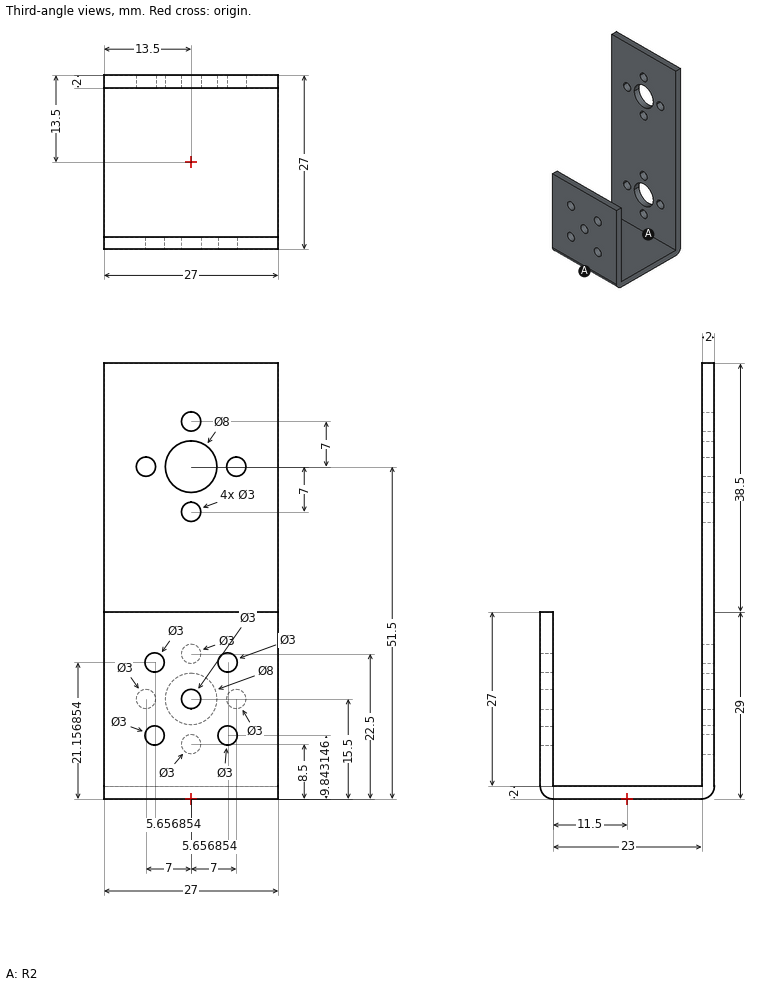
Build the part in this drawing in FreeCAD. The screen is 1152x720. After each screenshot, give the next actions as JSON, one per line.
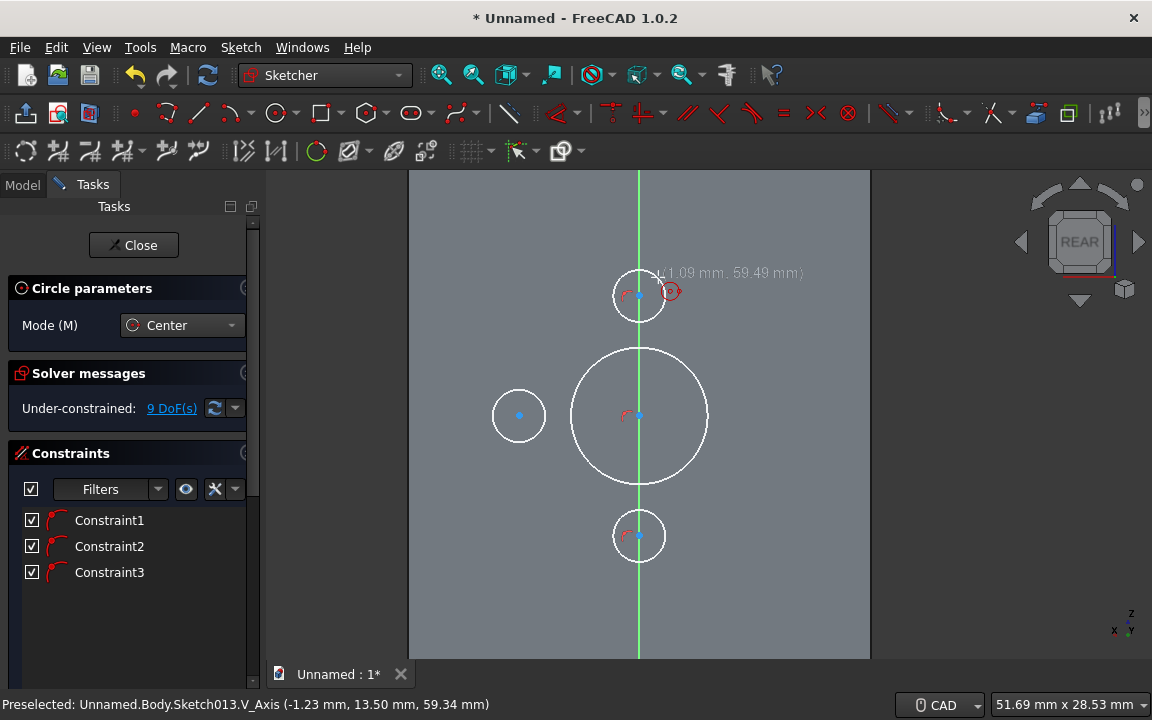
{"action": "left_click", "coordinate": [759, 415]}
{"action": "left_click", "coordinate": [777, 397]}
{"action": "key", "text": "Escape"}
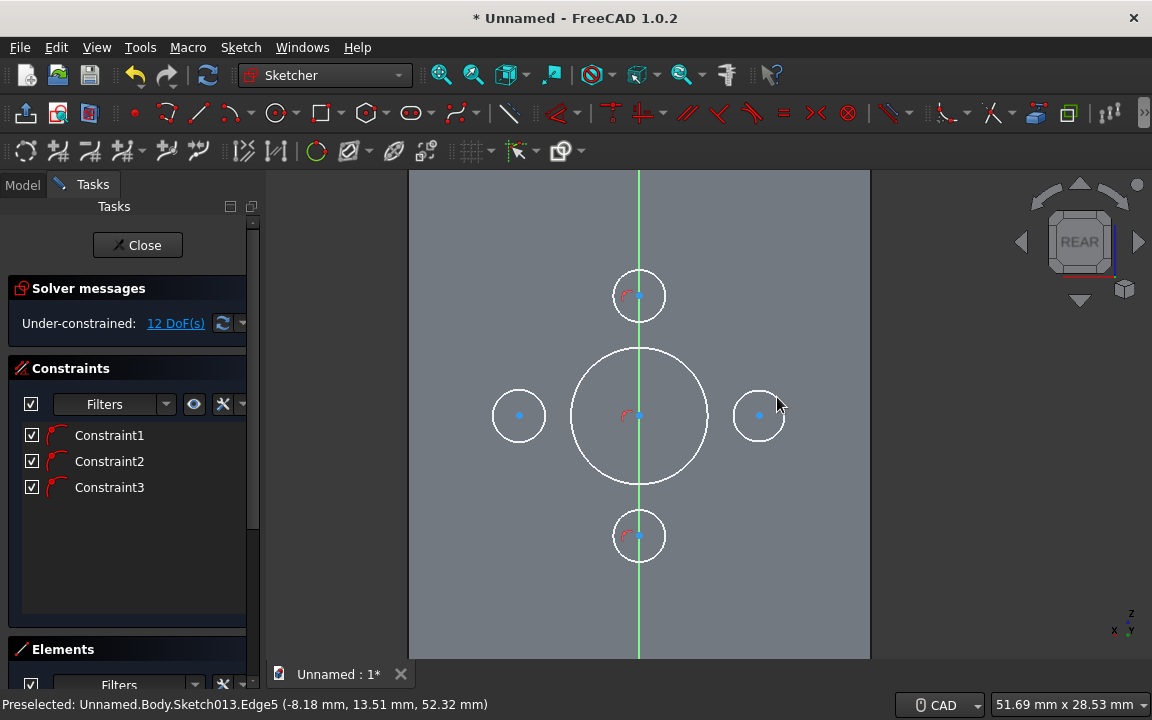
{"action": "left_click", "coordinate": [658, 518]}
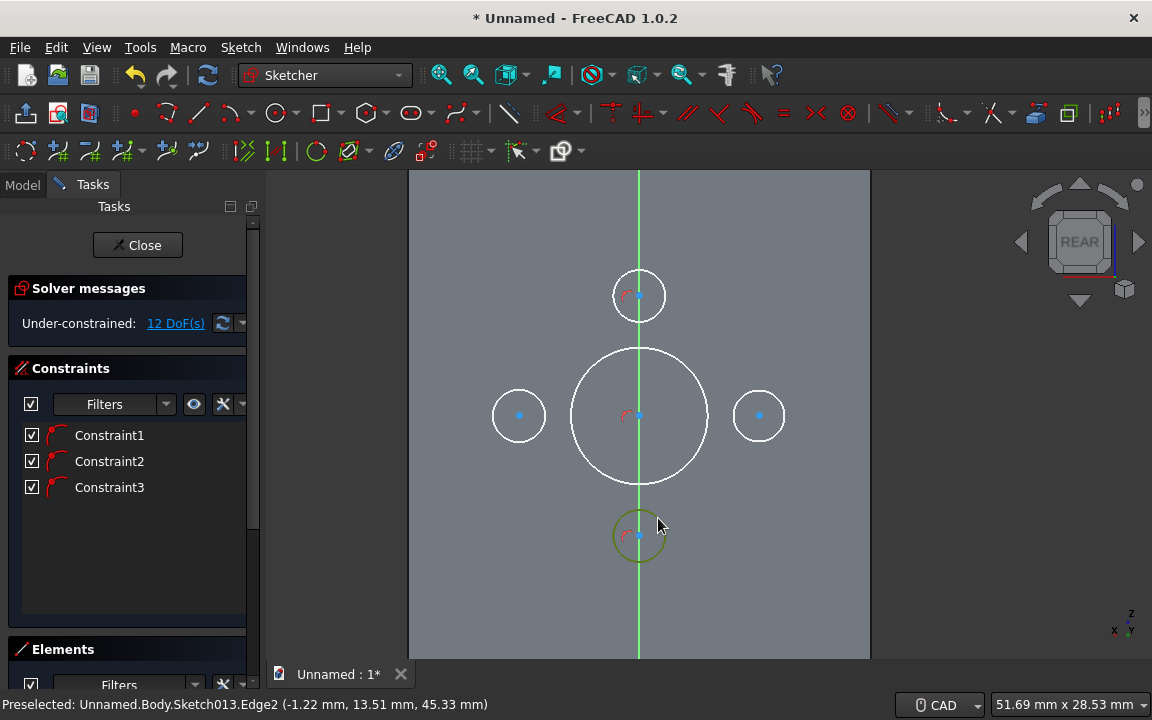
{"action": "left_click", "coordinate": [537, 397]}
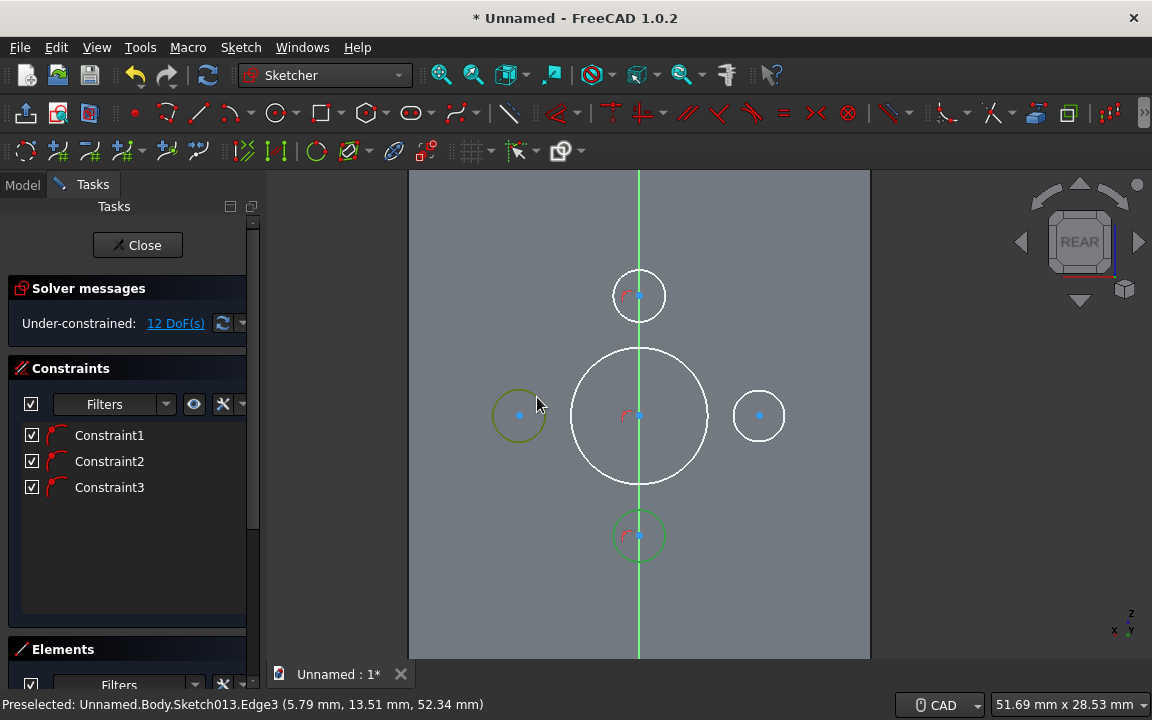
{"action": "left_click", "coordinate": [658, 278]}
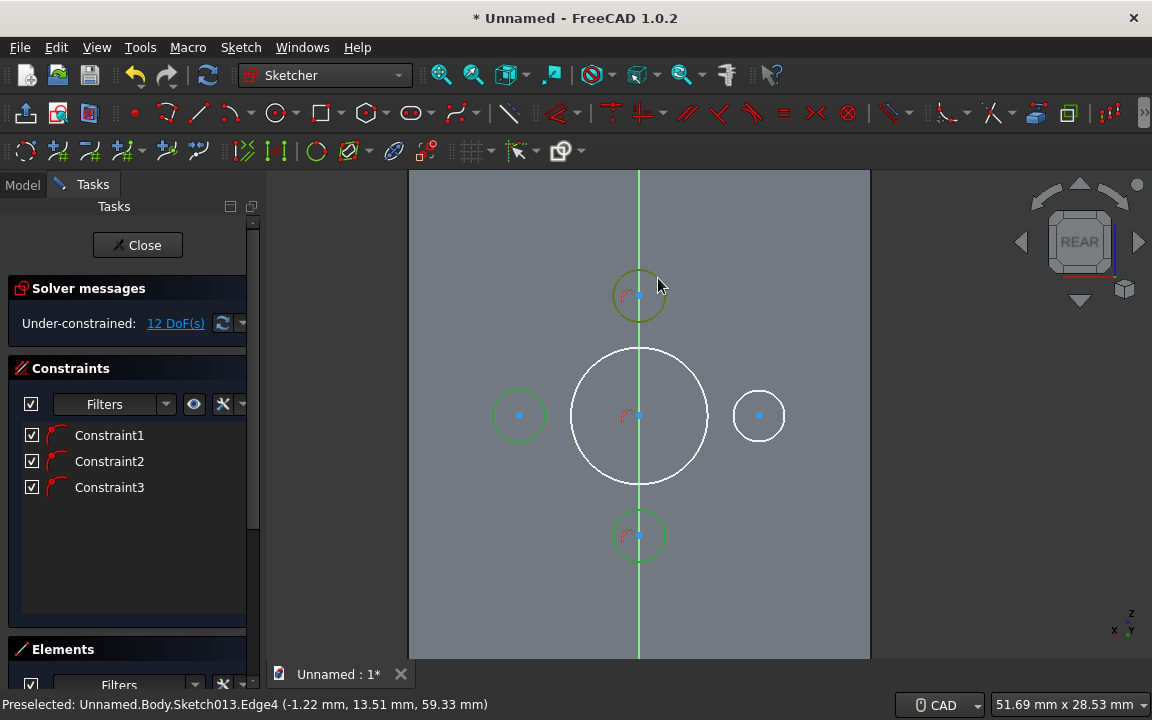
{"action": "left_click", "coordinate": [777, 398]}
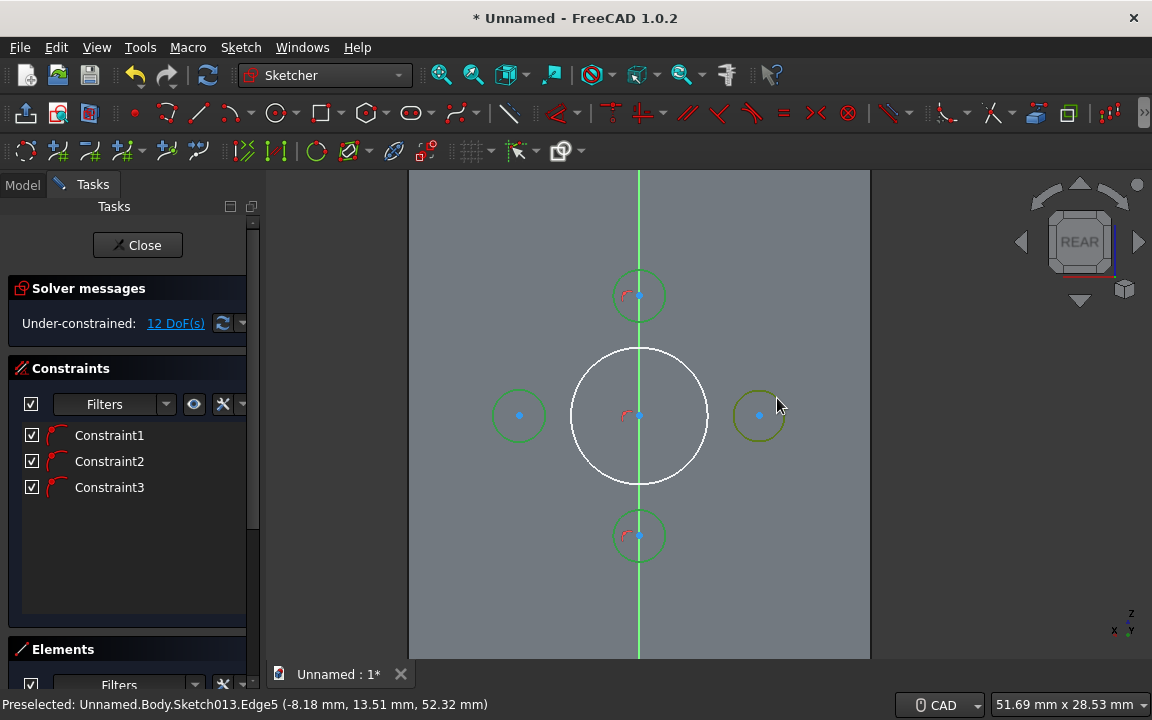
{"action": "key", "text": "e"}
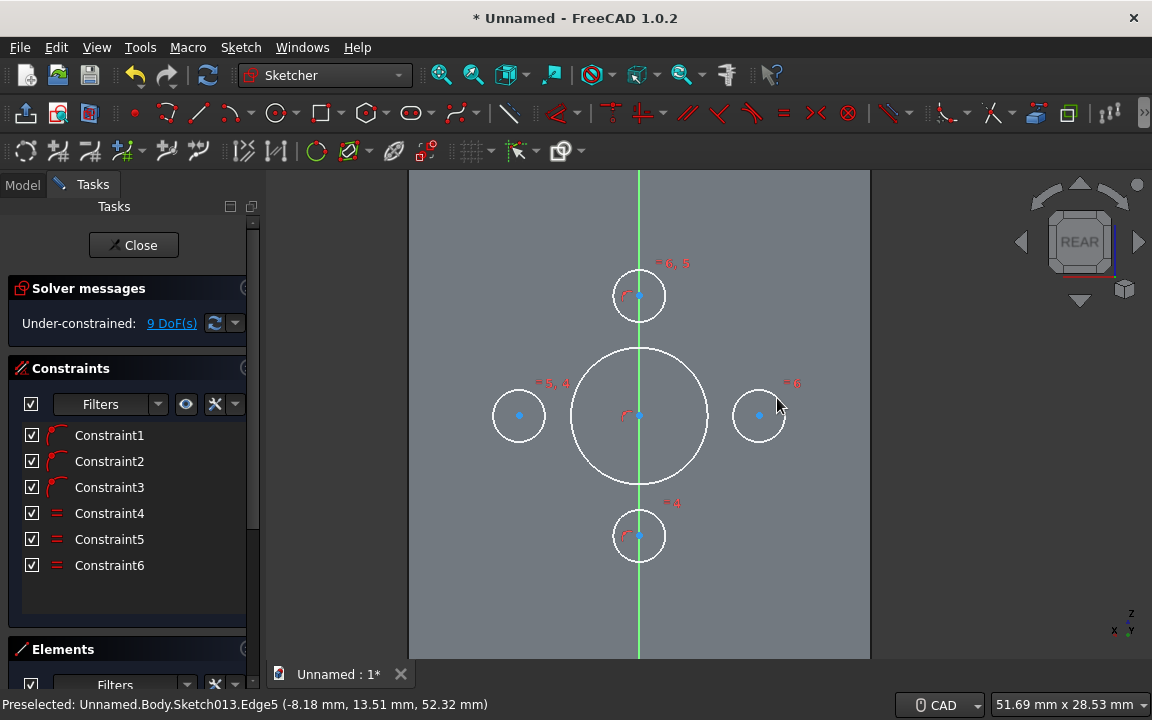
{"action": "left_click", "coordinate": [639, 416]}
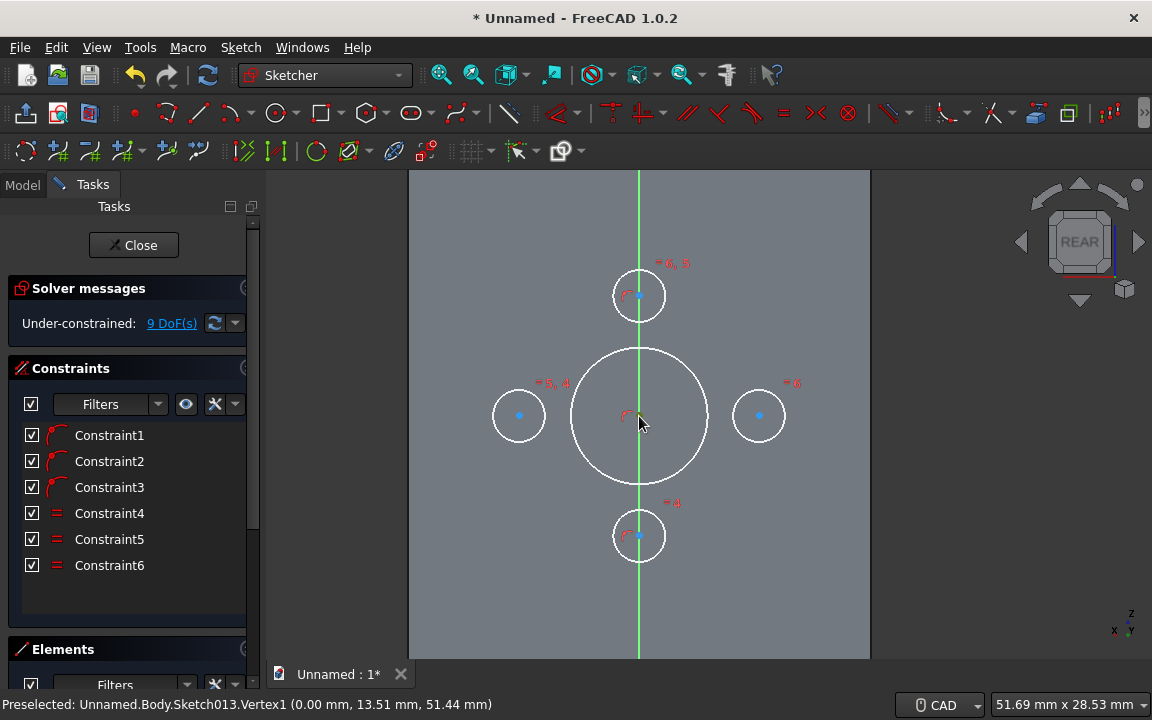
{"action": "left_click", "coordinate": [519, 416]}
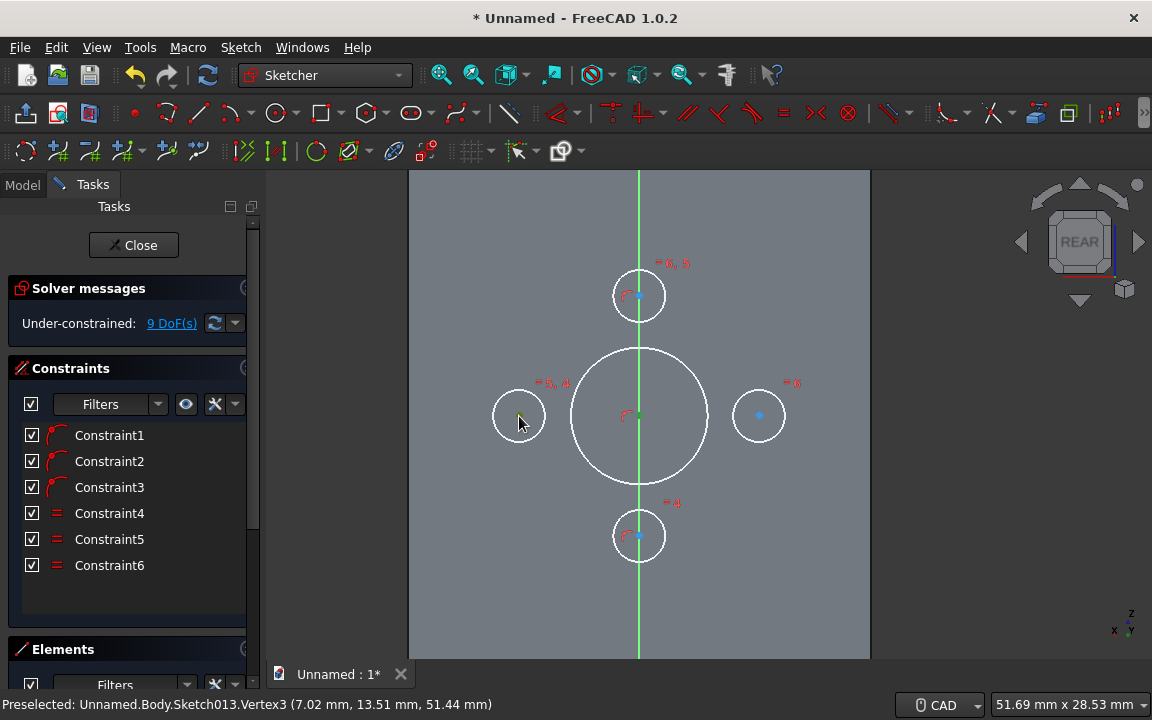
{"action": "key", "text": "h"}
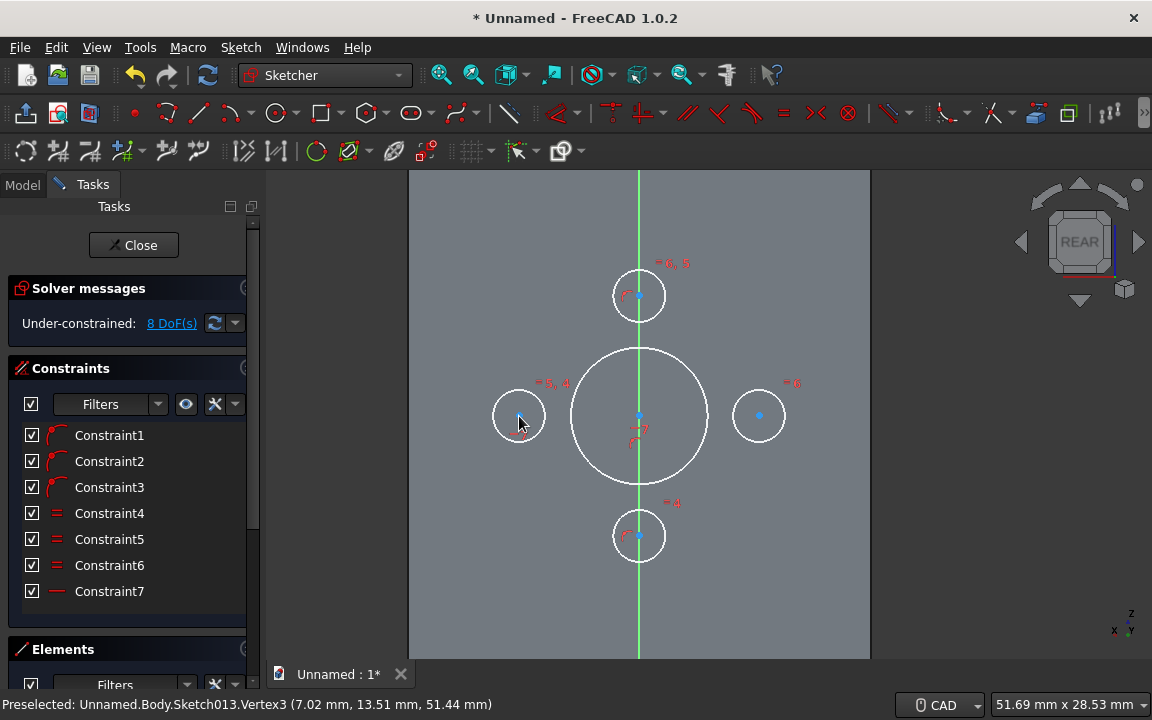
{"action": "left_click", "coordinate": [639, 416]}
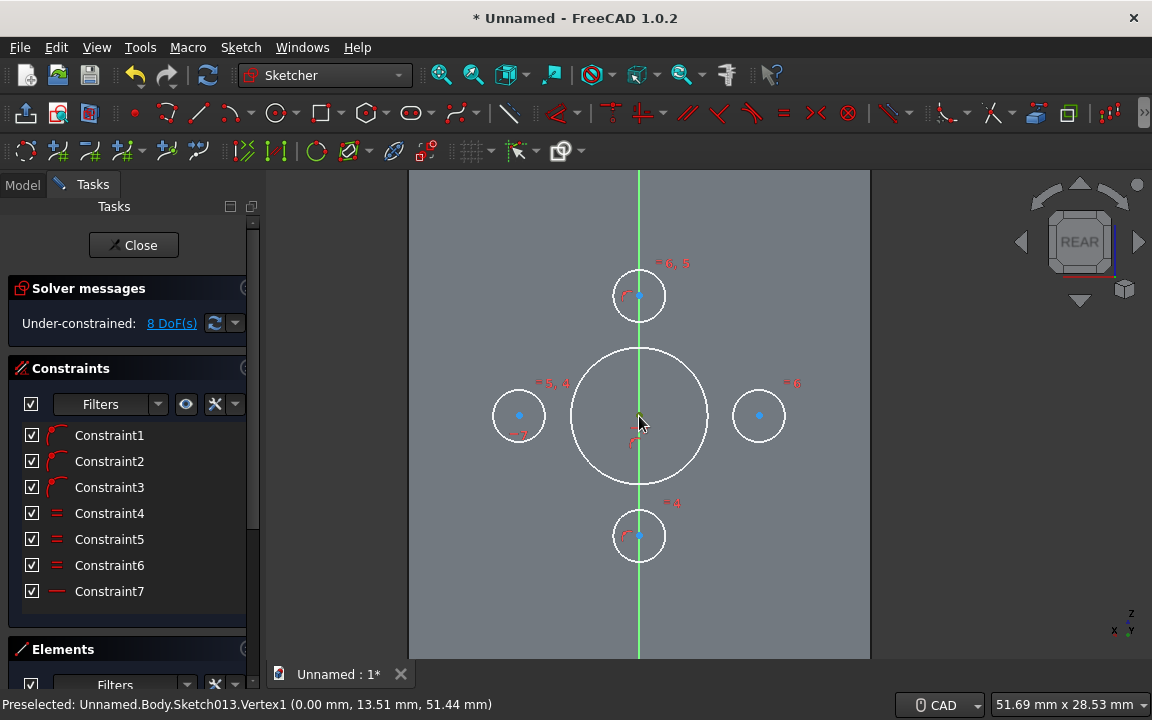
{"action": "left_click", "coordinate": [759, 416]}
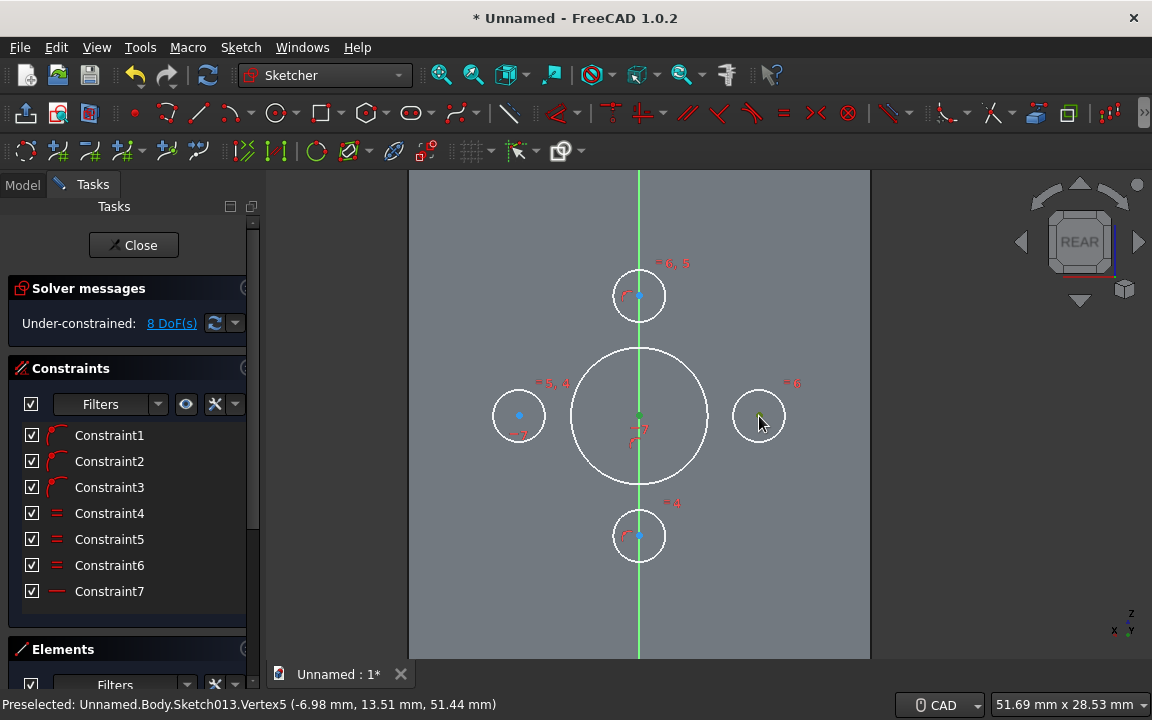
{"action": "key", "text": "h"}